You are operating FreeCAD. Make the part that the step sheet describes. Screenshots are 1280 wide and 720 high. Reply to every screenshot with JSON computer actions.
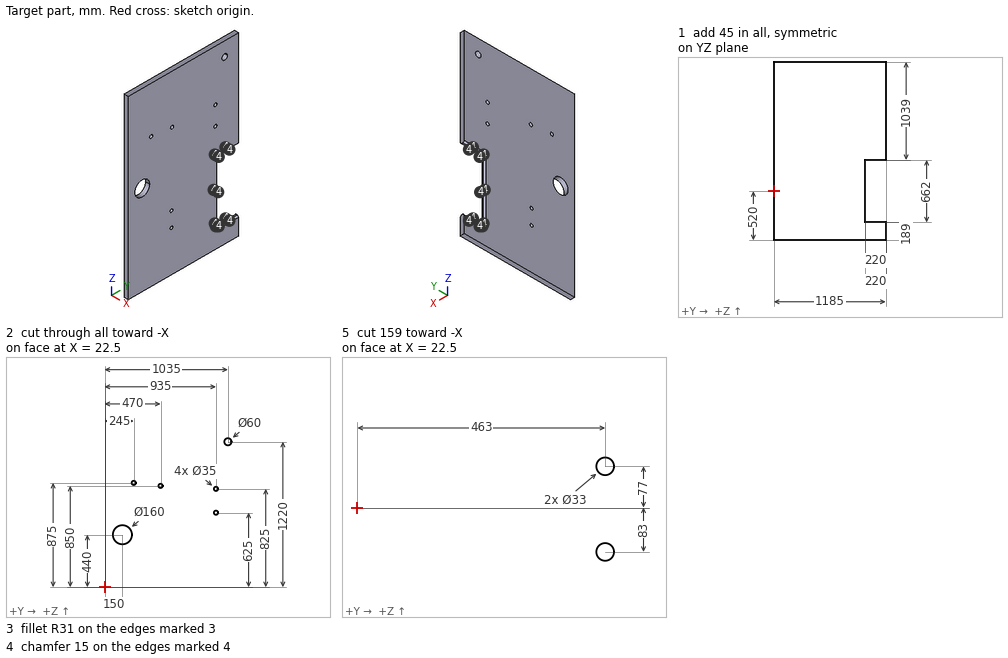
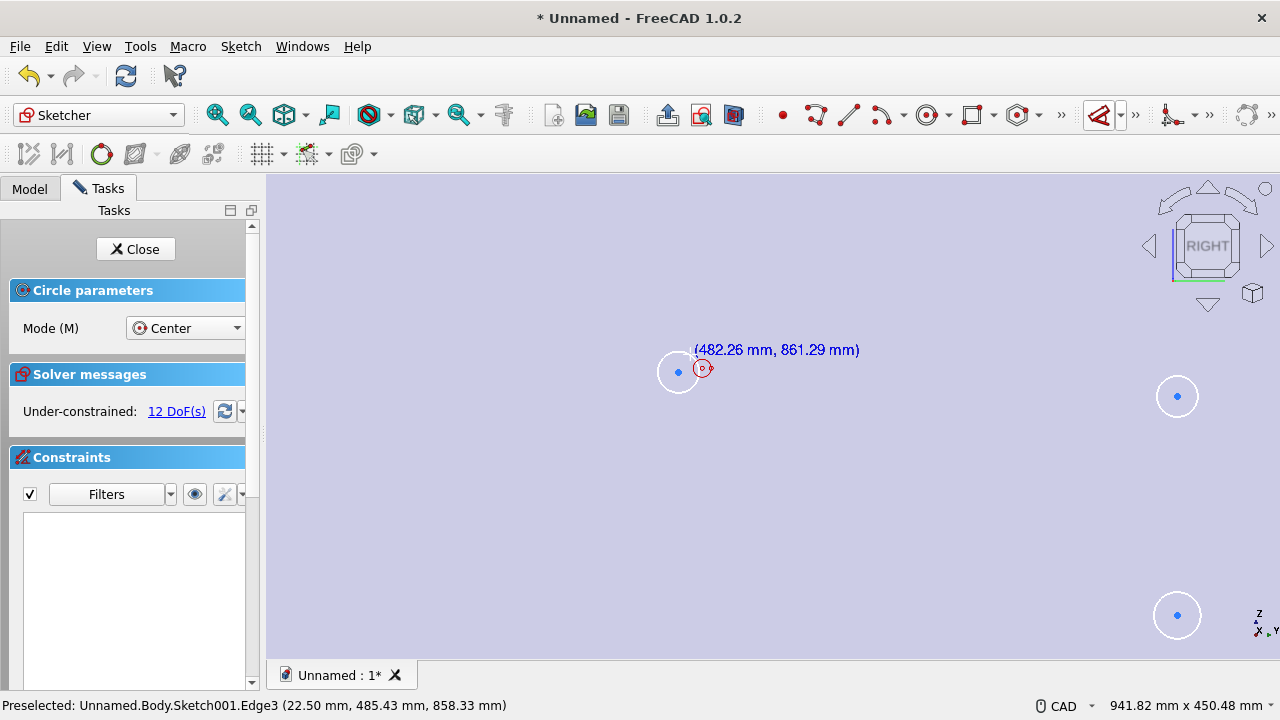
{"action": "scroll", "coordinate": [692, 353], "scroll_direction": "down", "scroll_amount": 7}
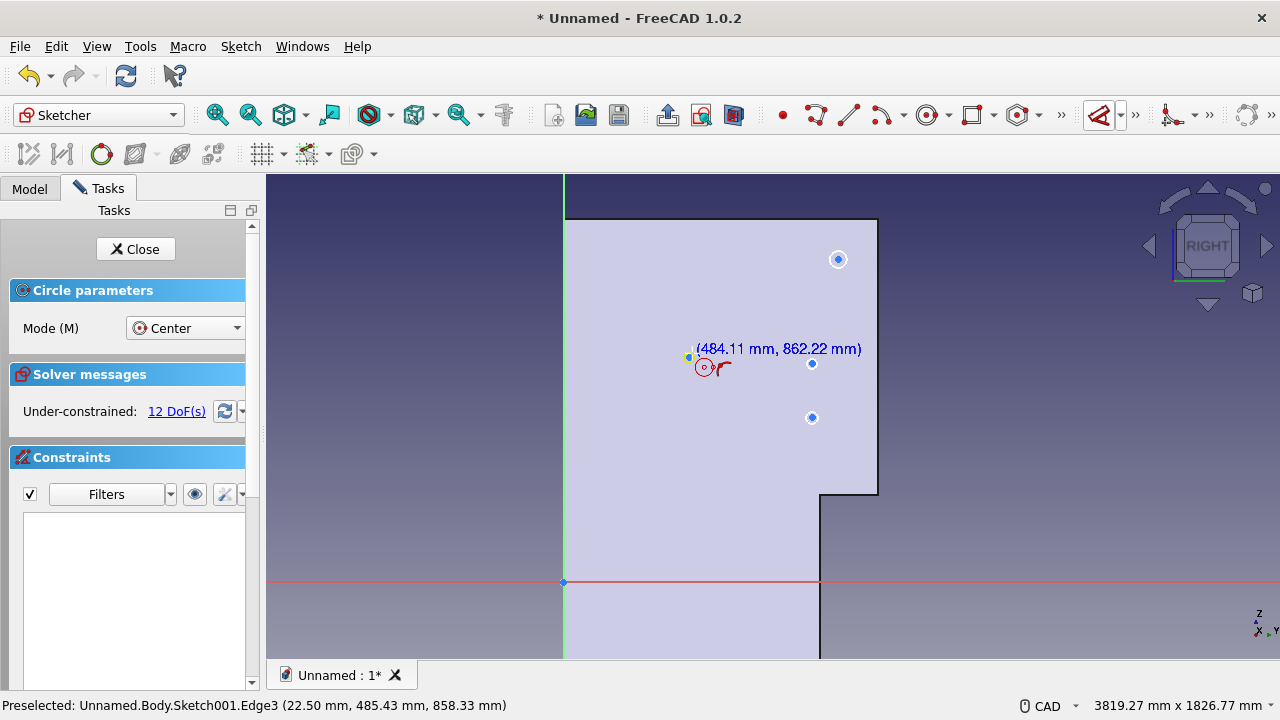
{"action": "left_click", "coordinate": [629, 350]}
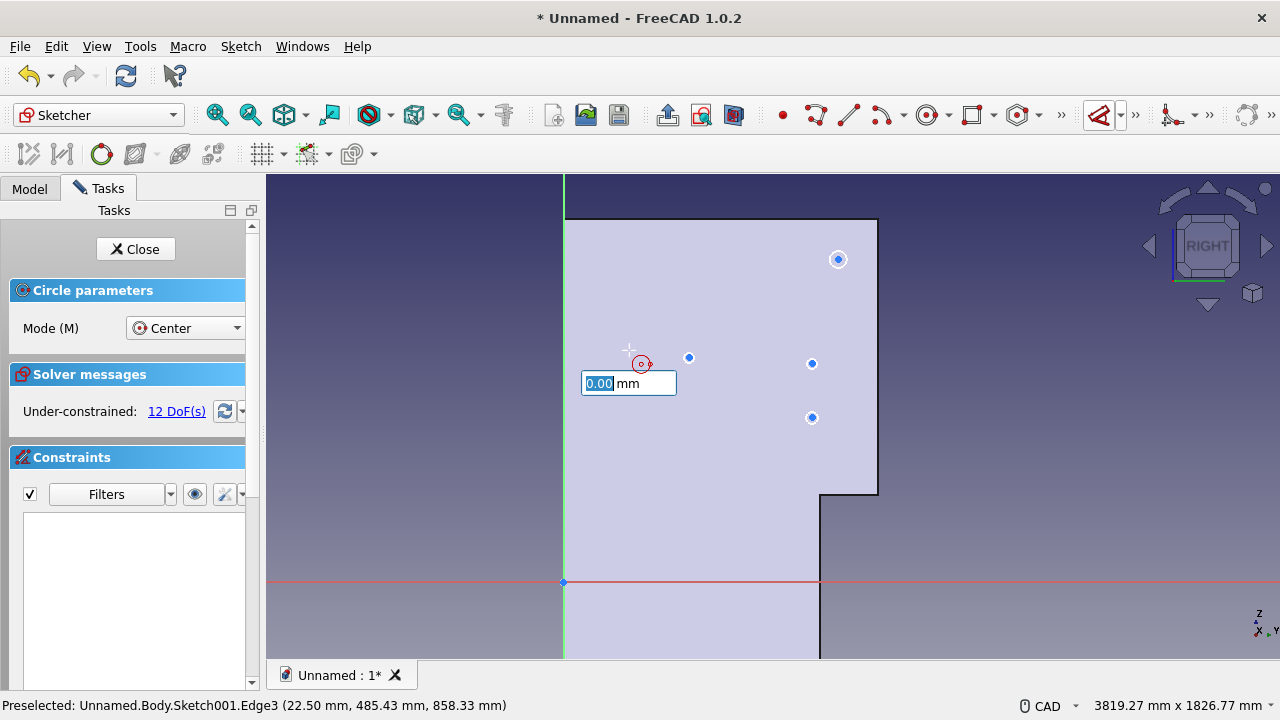
{"action": "scroll", "coordinate": [632, 347], "scroll_direction": "up", "scroll_amount": 7}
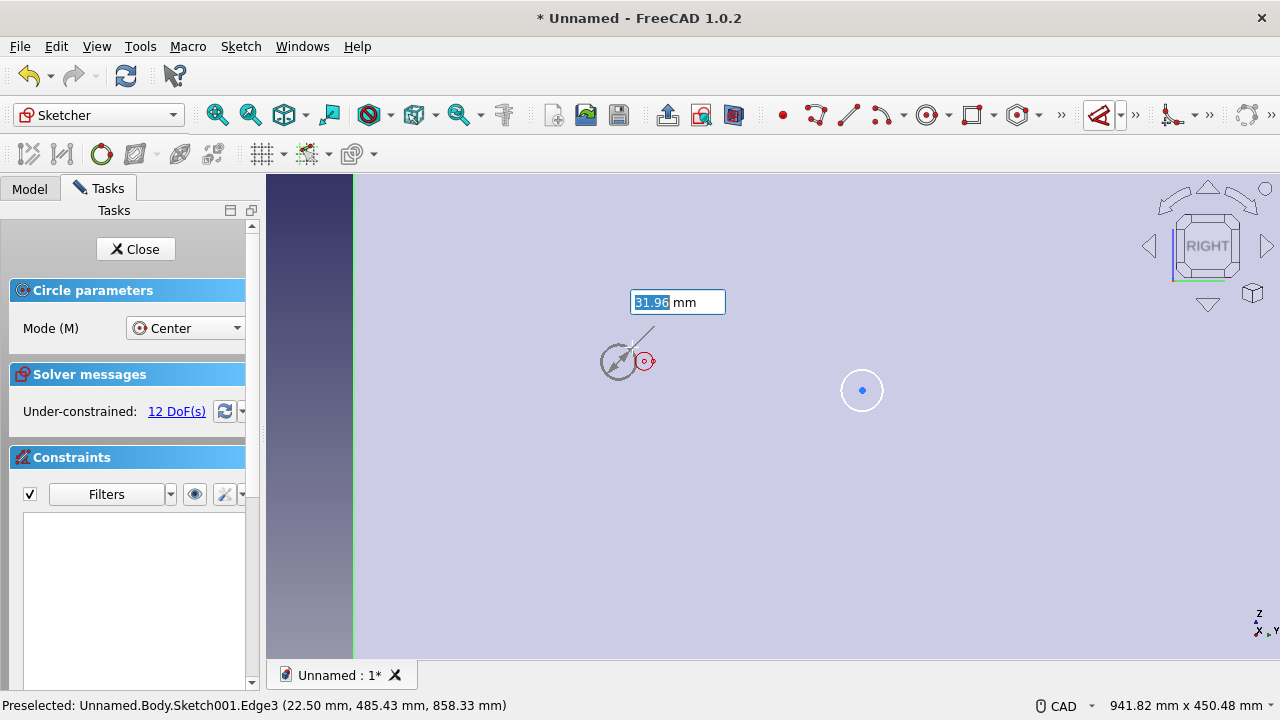
{"action": "left_click", "coordinate": [631, 345]}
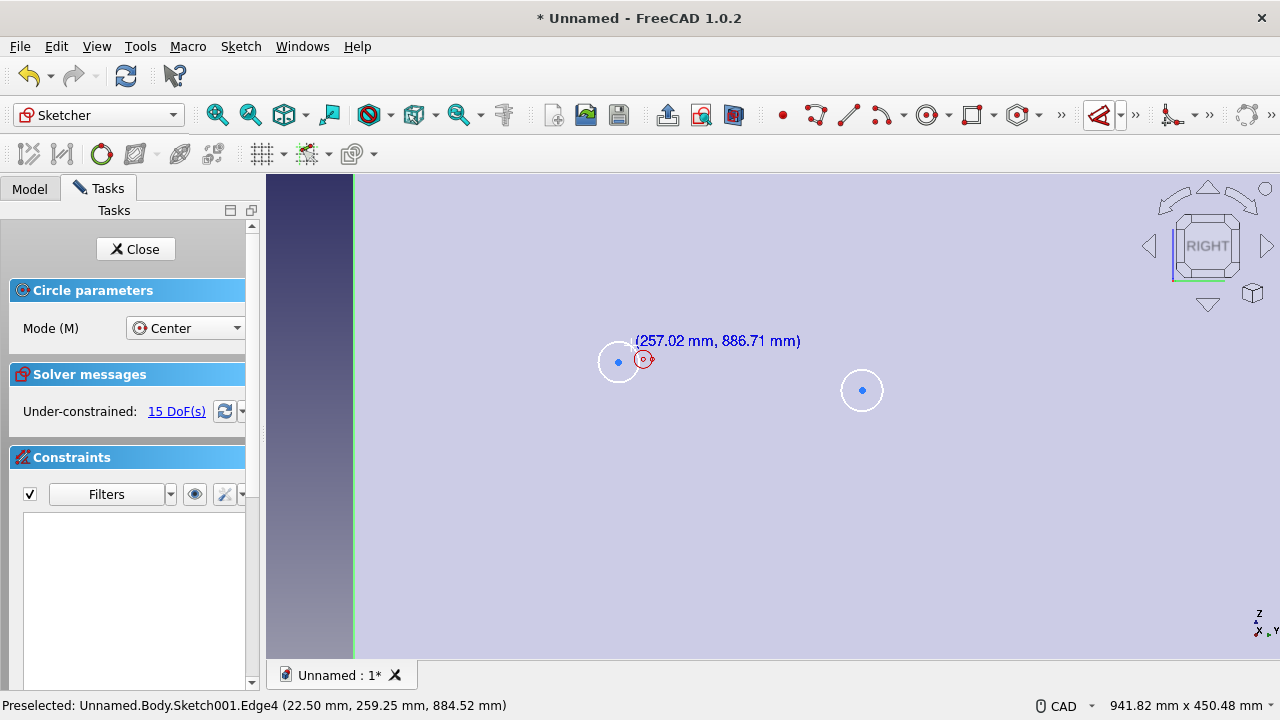
{"action": "scroll", "coordinate": [631, 347], "scroll_direction": "down", "scroll_amount": 7}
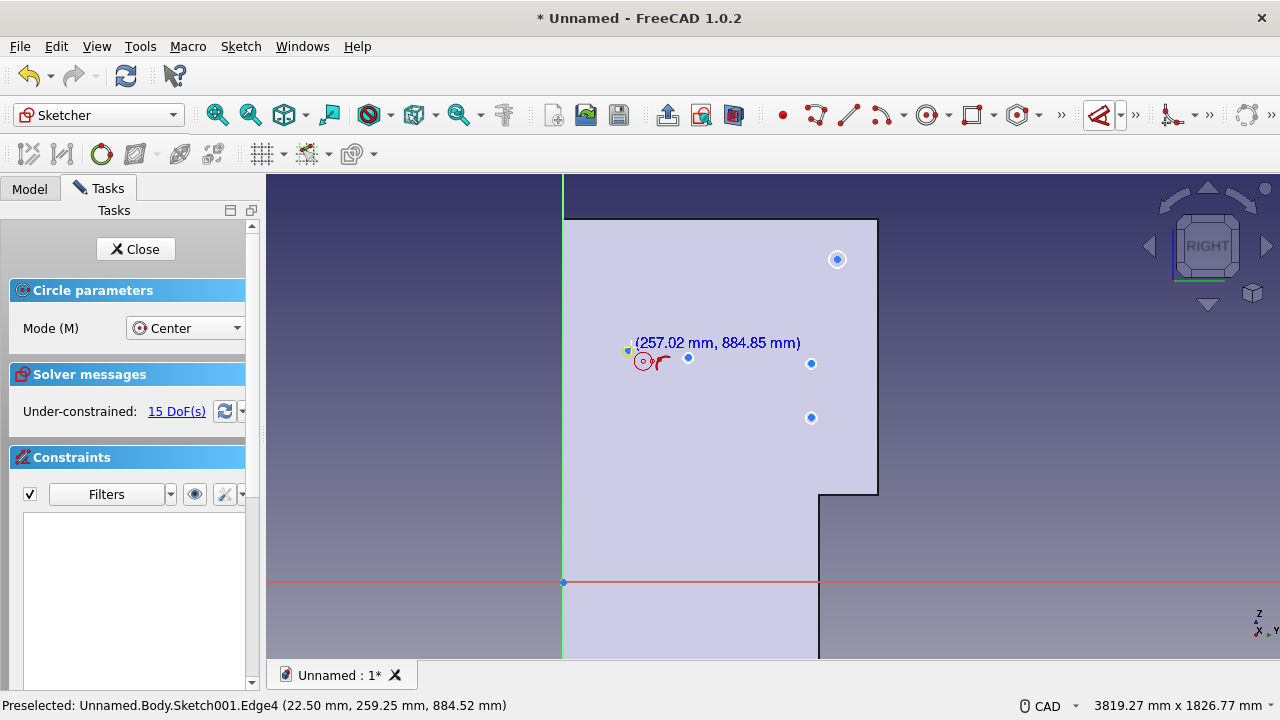
{"action": "left_click", "coordinate": [603, 466]}
{"action": "left_click", "coordinate": [618, 451]}
{"action": "key", "text": "Escape"}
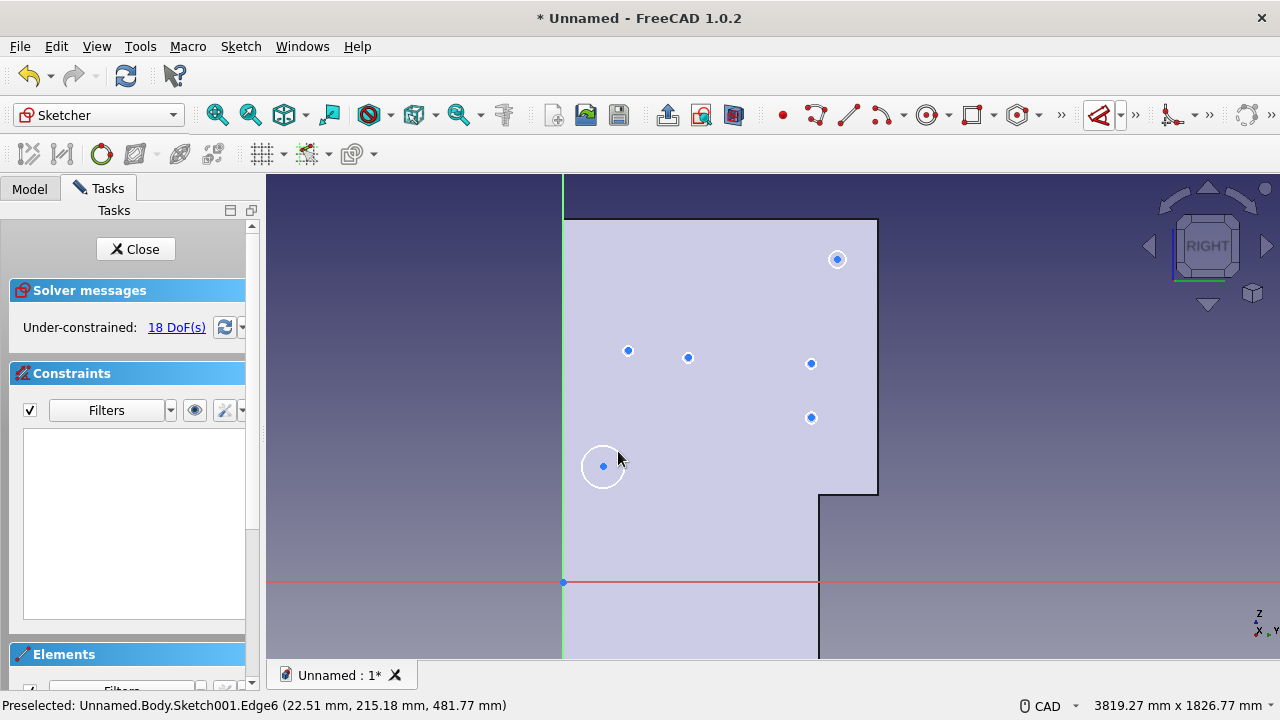
{"action": "scroll", "coordinate": [815, 360], "scroll_direction": "up", "scroll_amount": 6}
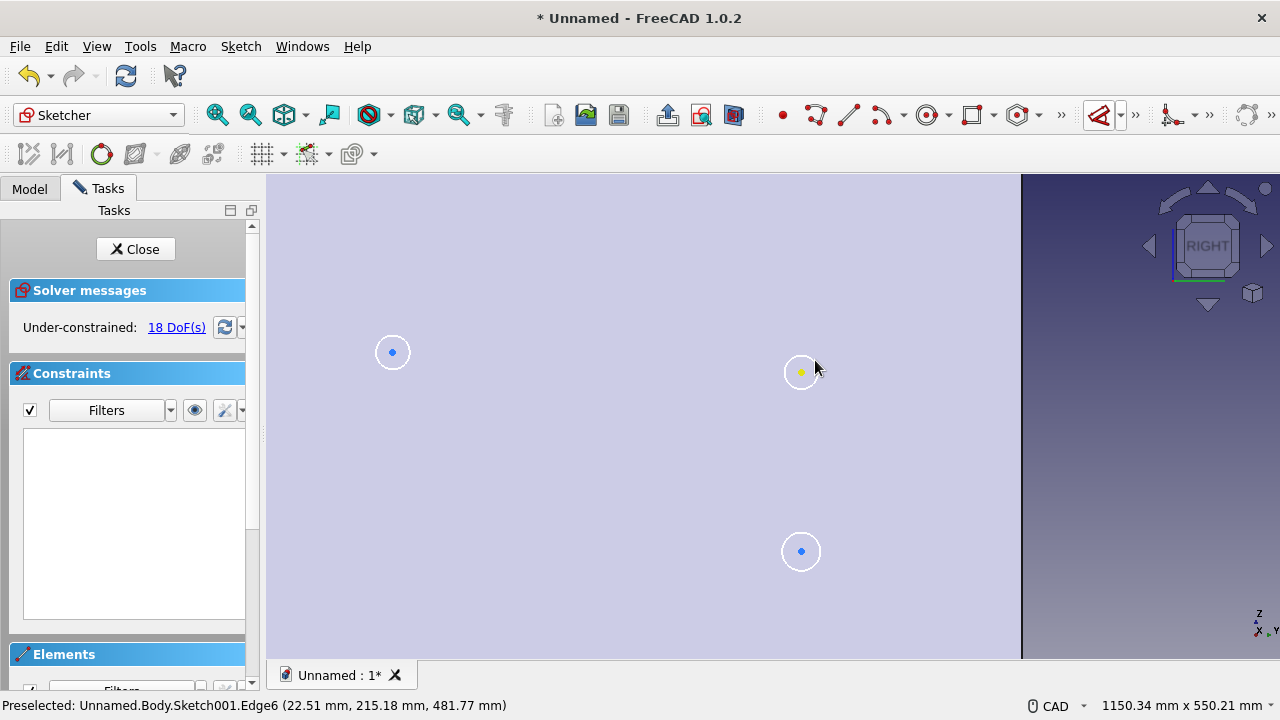
{"action": "left_click", "coordinate": [813, 361]}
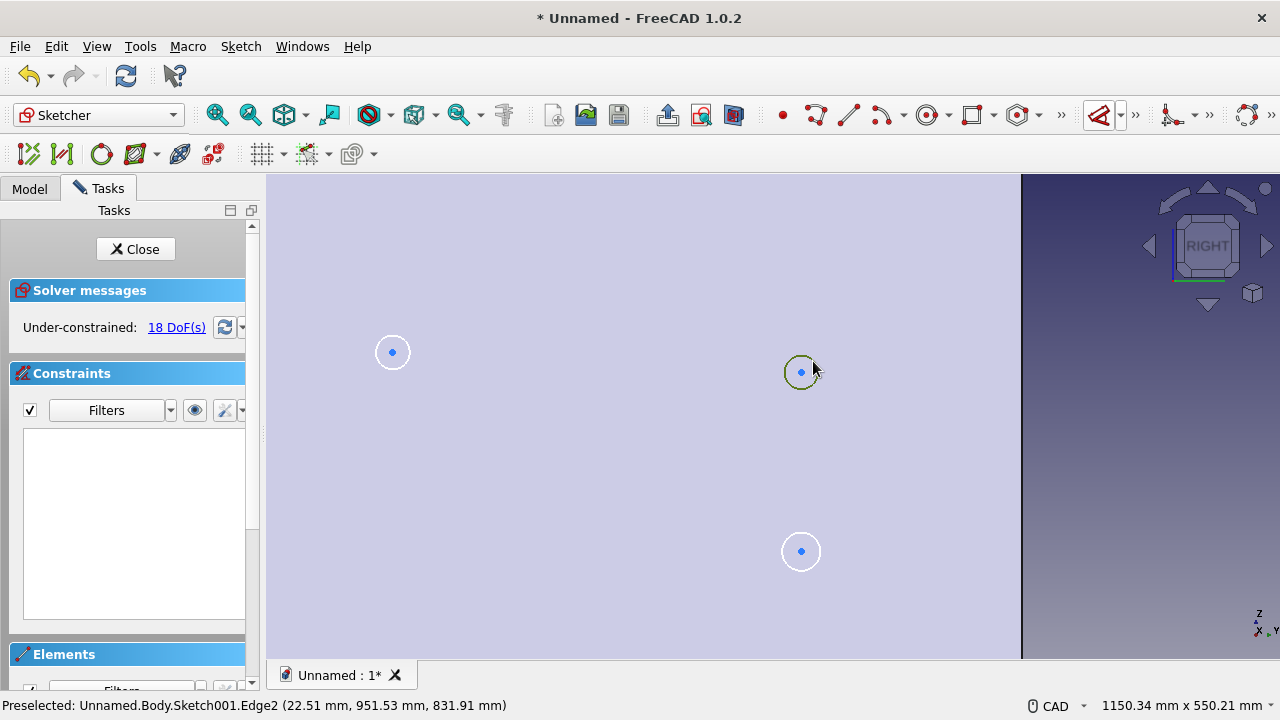
{"action": "left_click", "coordinate": [815, 538]}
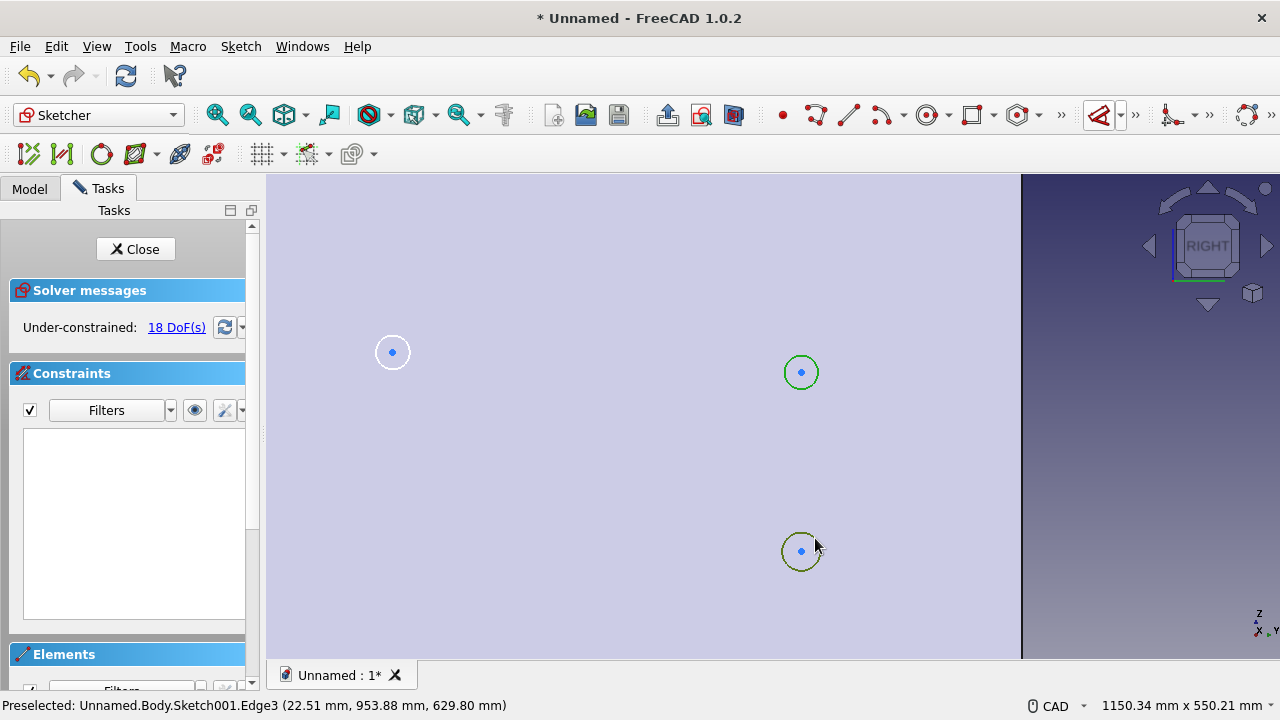
{"action": "left_click", "coordinate": [405, 340]}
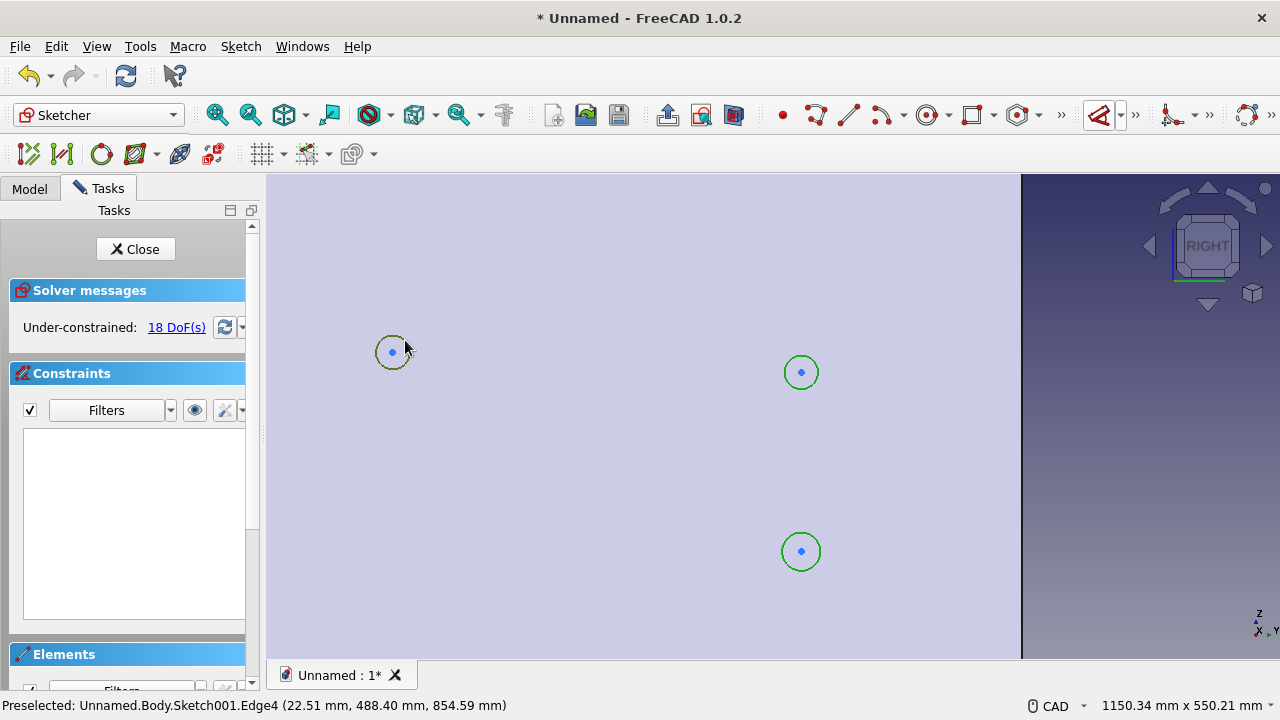
{"action": "scroll", "coordinate": [816, 360], "scroll_direction": "down", "scroll_amount": 6}